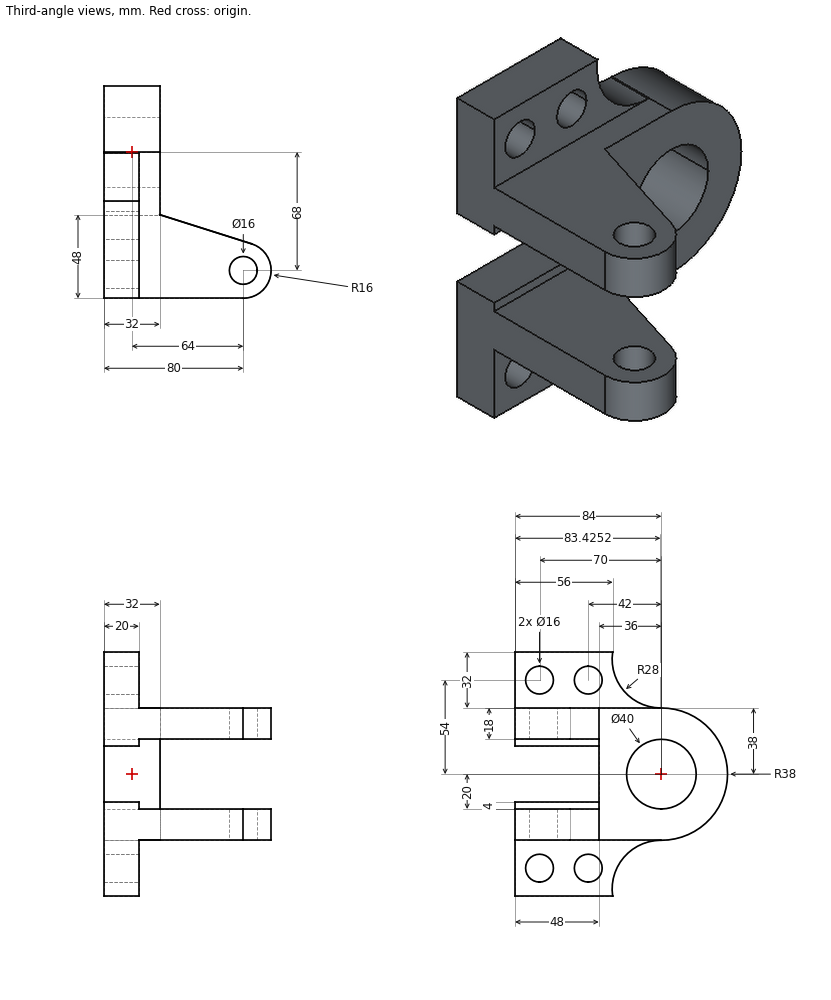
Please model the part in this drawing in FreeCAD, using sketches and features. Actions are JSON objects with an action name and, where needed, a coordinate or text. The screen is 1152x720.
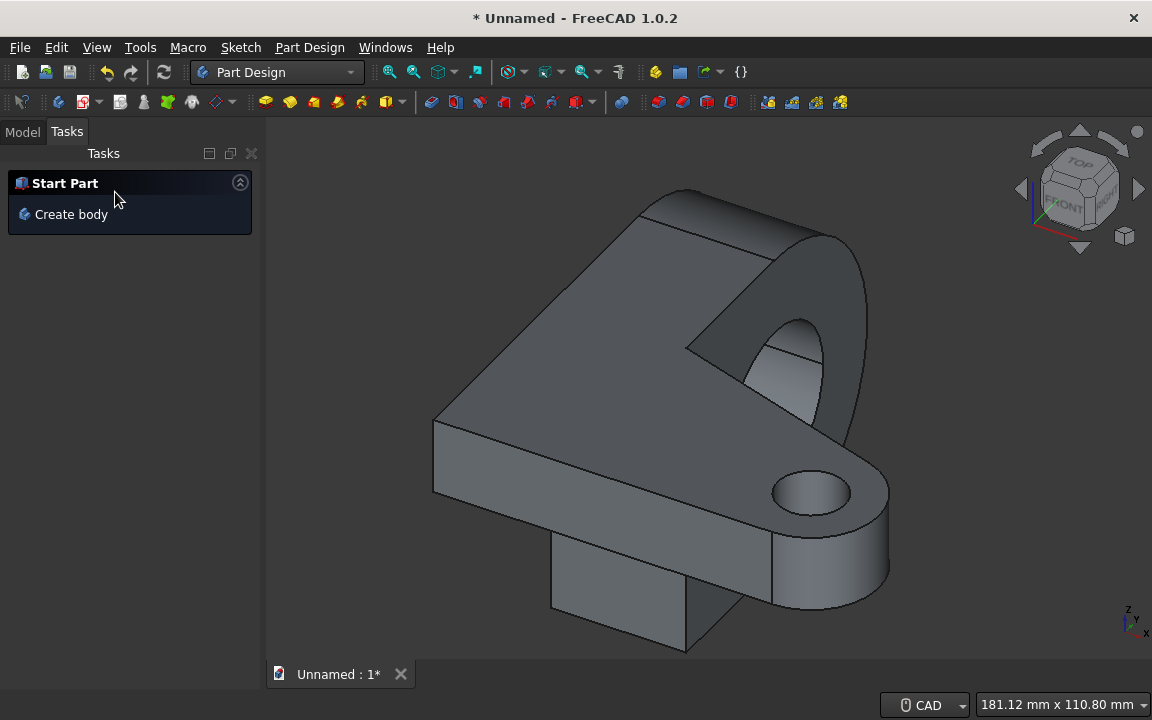
{"action": "left_click", "coordinate": [390, 72]}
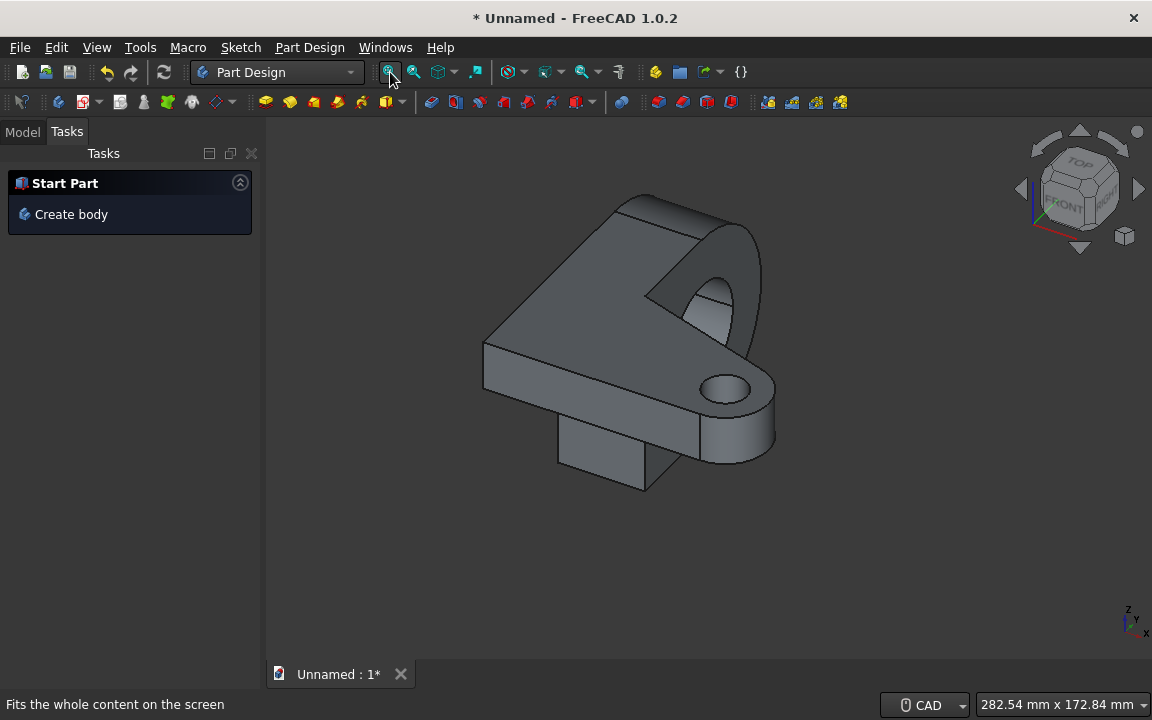
{"action": "left_click", "coordinate": [23, 131]}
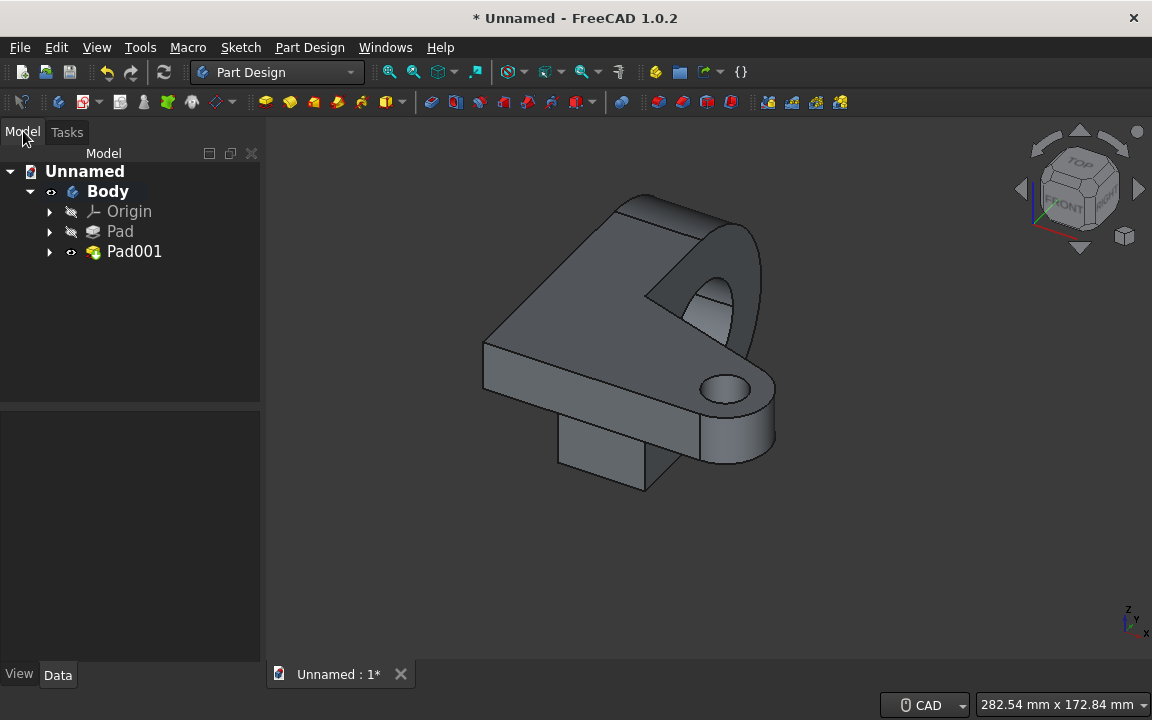
{"action": "left_click", "coordinate": [116, 252]}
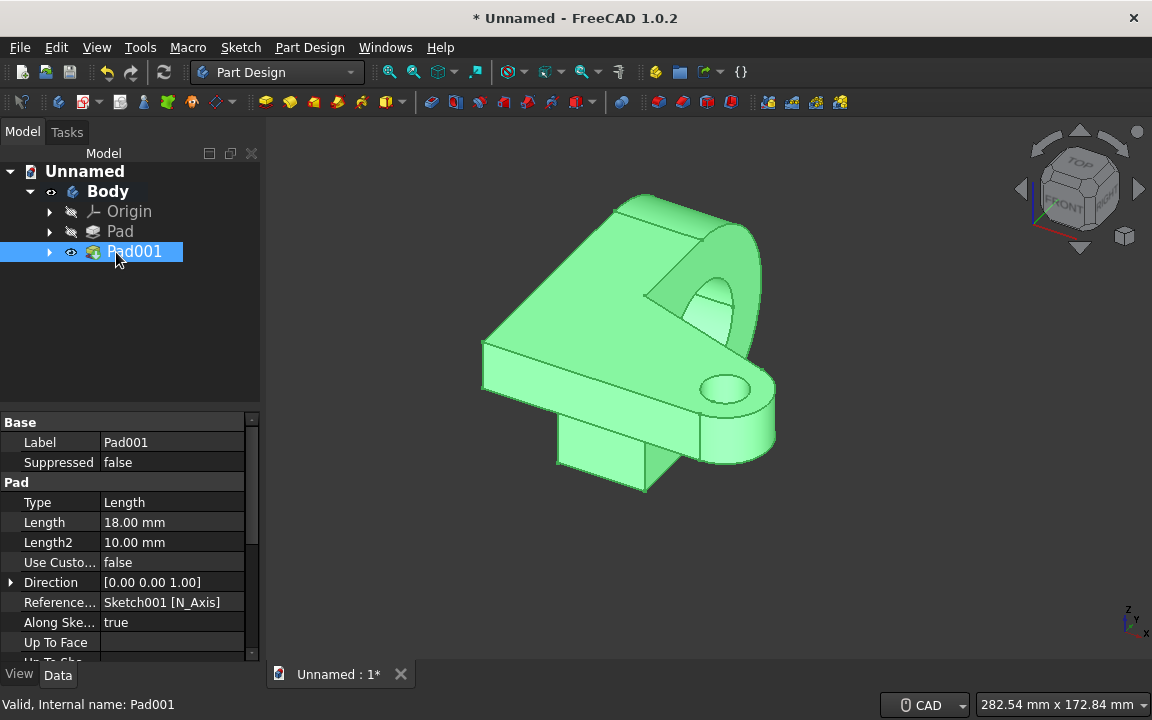
{"action": "left_click", "coordinate": [768, 102]}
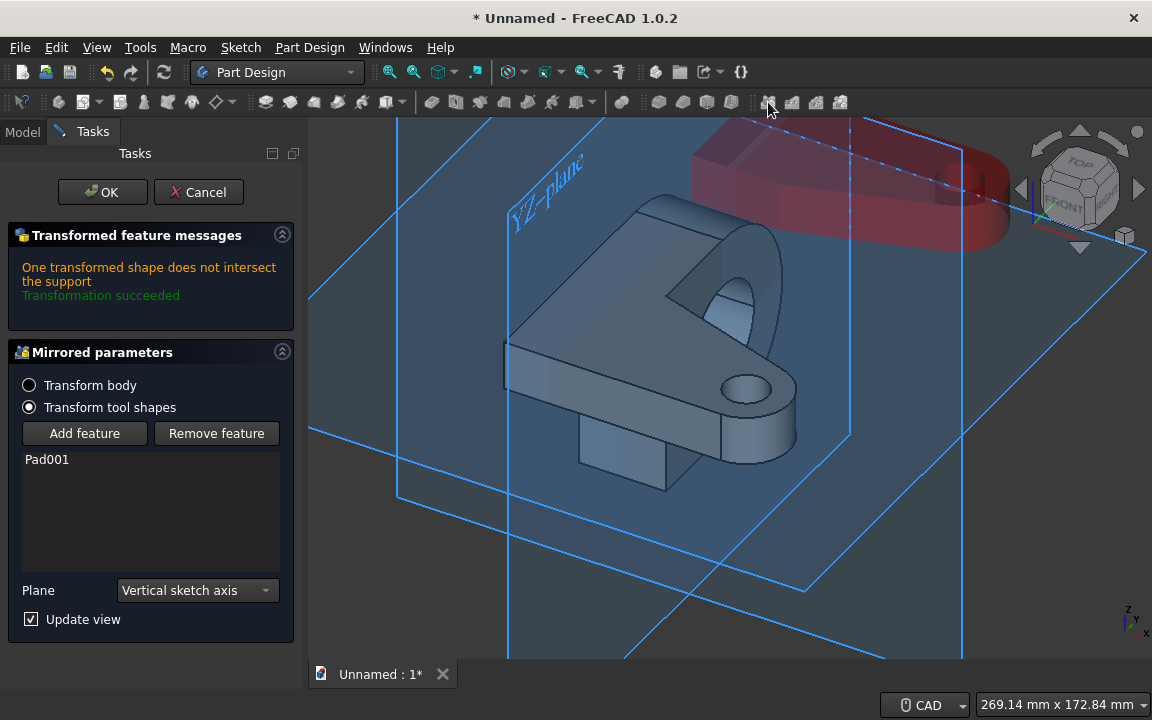
{"action": "left_click", "coordinate": [198, 590]}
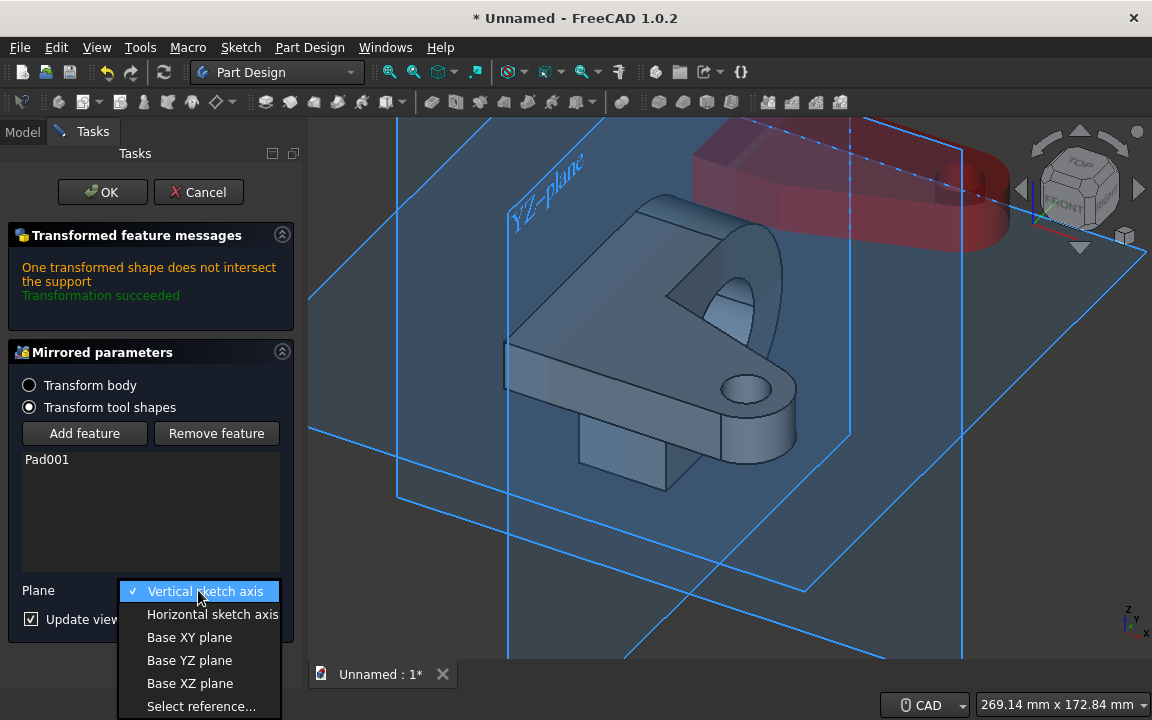
{"action": "left_click", "coordinate": [198, 638]}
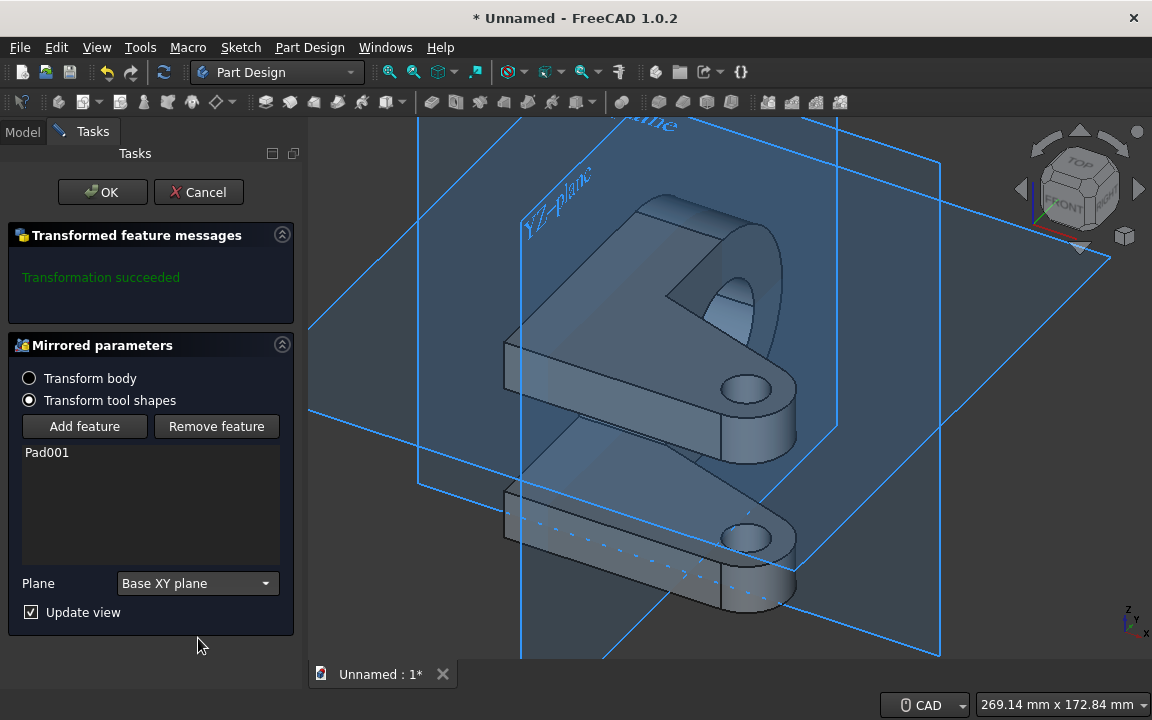
{"action": "left_click", "coordinate": [103, 192]}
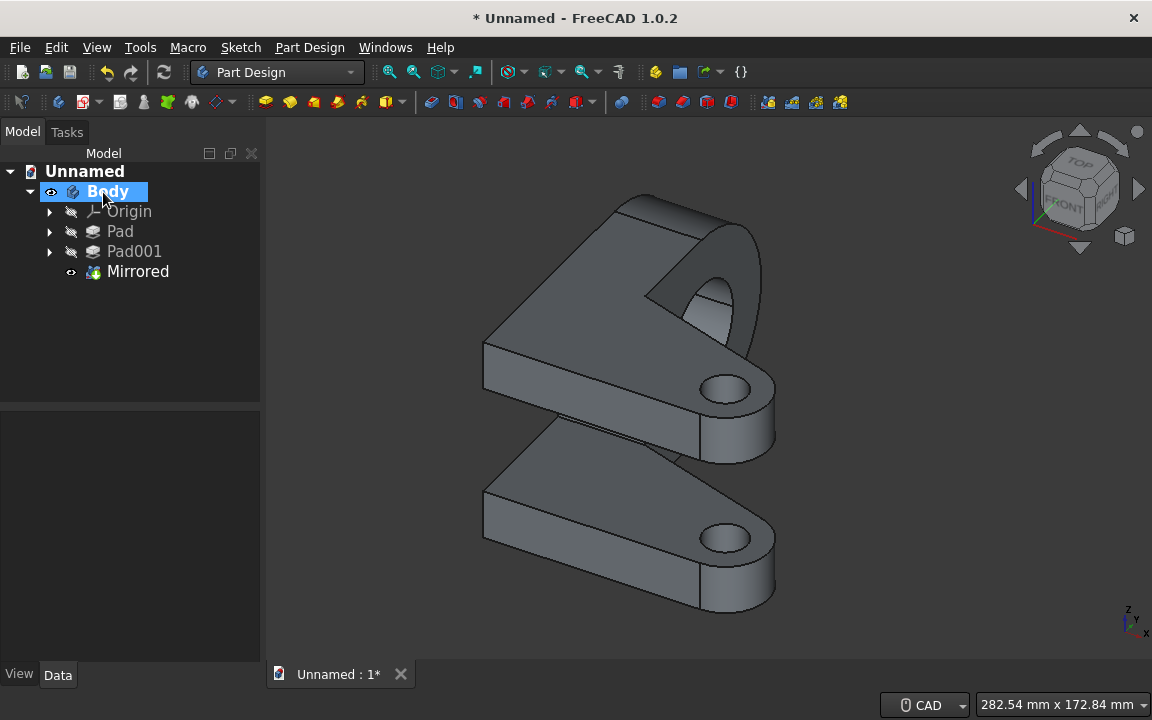
{"action": "key", "text": "6"}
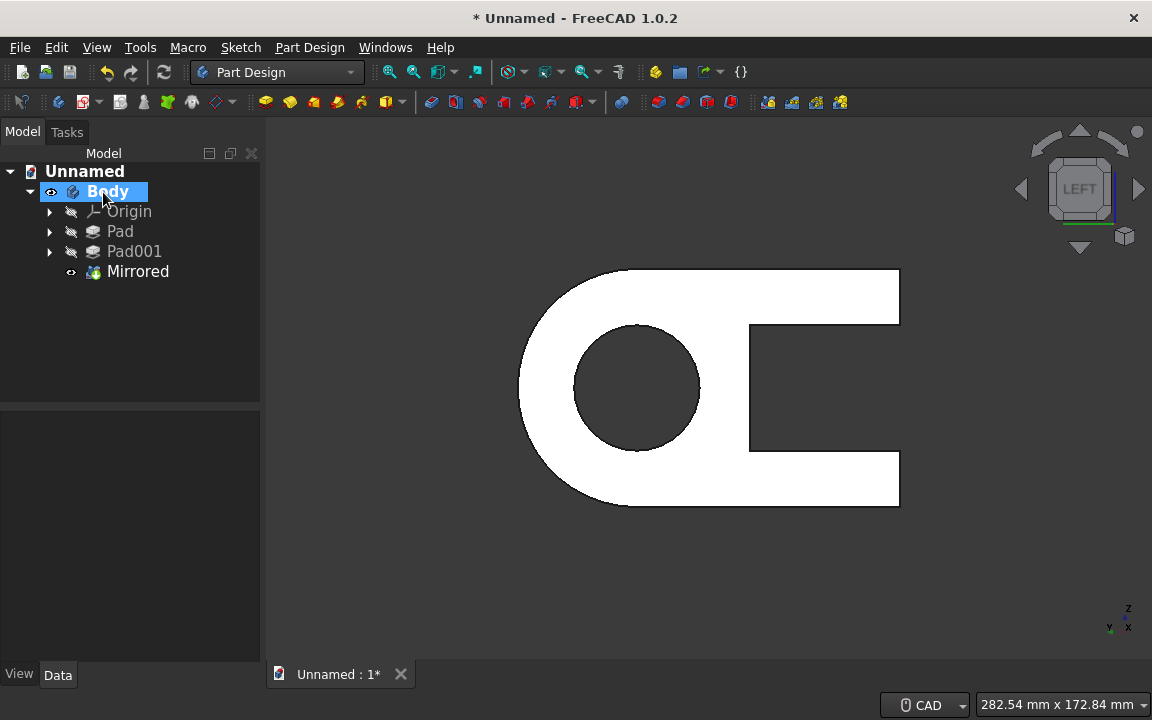
{"action": "left_click", "coordinate": [390, 72]}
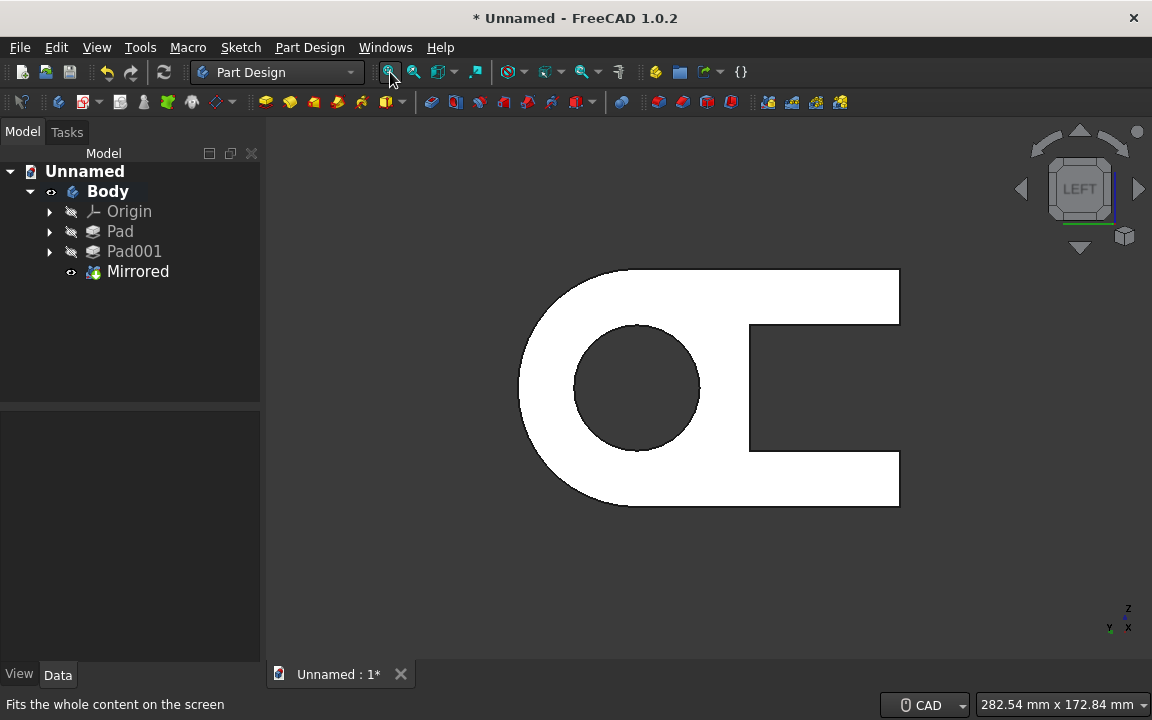
{"action": "left_click", "coordinate": [709, 319]}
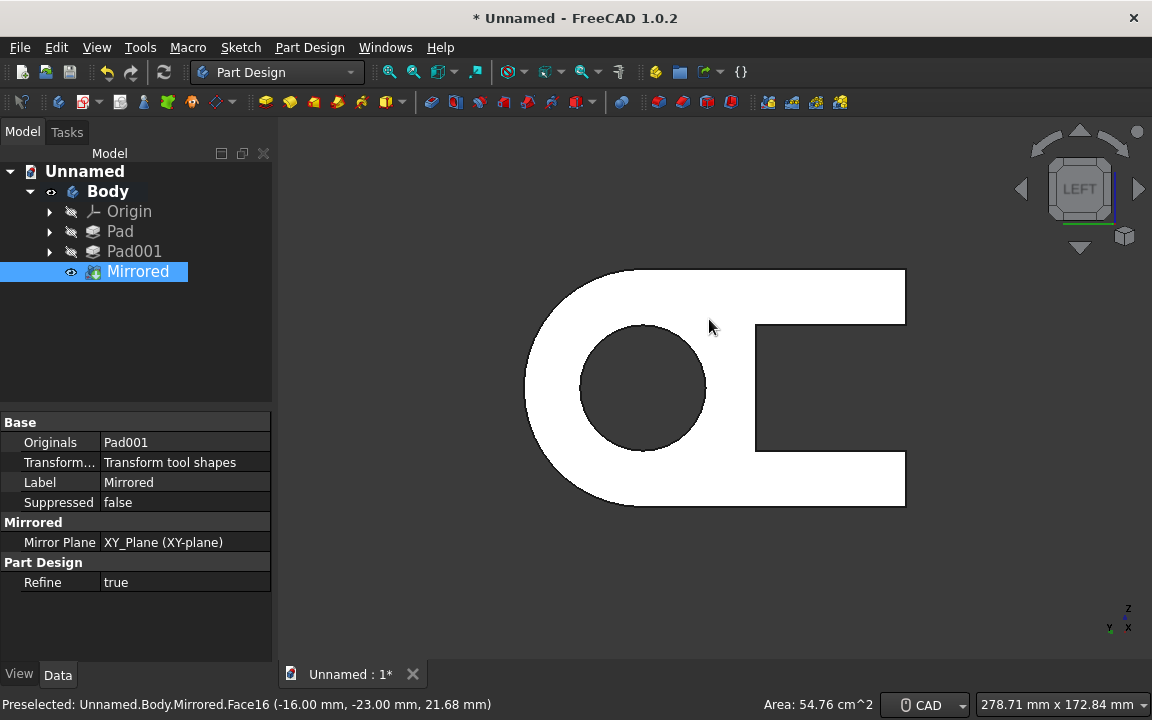
{"action": "left_click", "coordinate": [84, 102]}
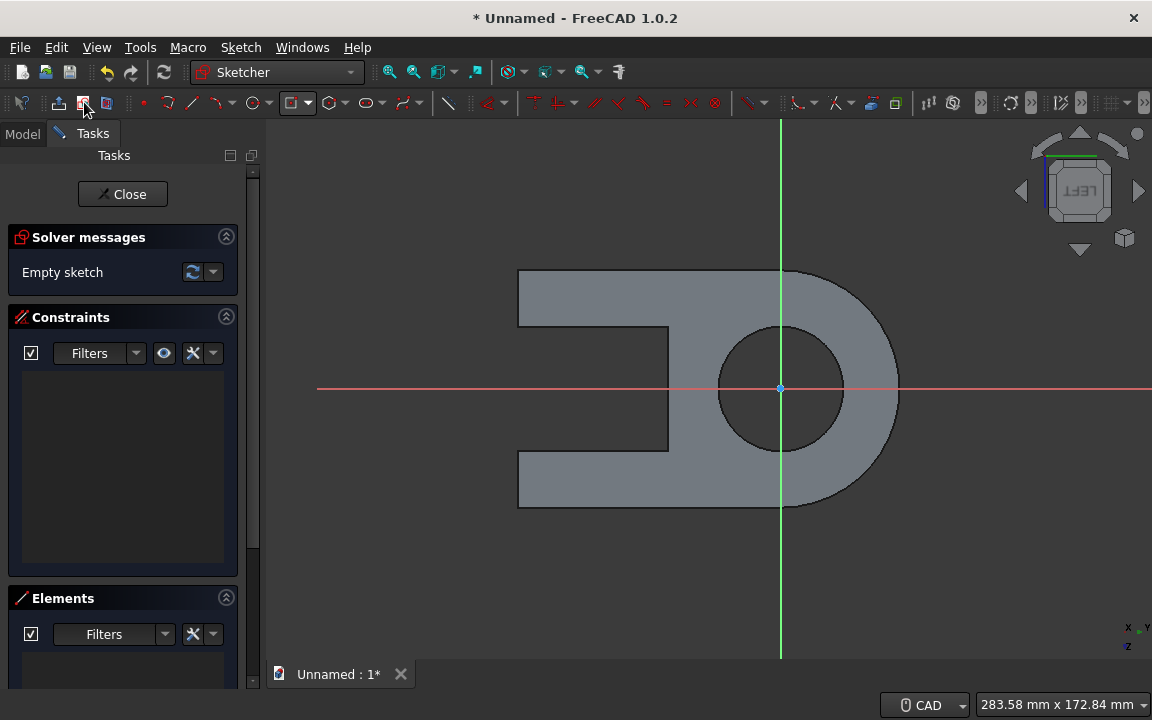
{"action": "scroll", "coordinate": [668, 631], "scroll_direction": "up", "scroll_amount": 2}